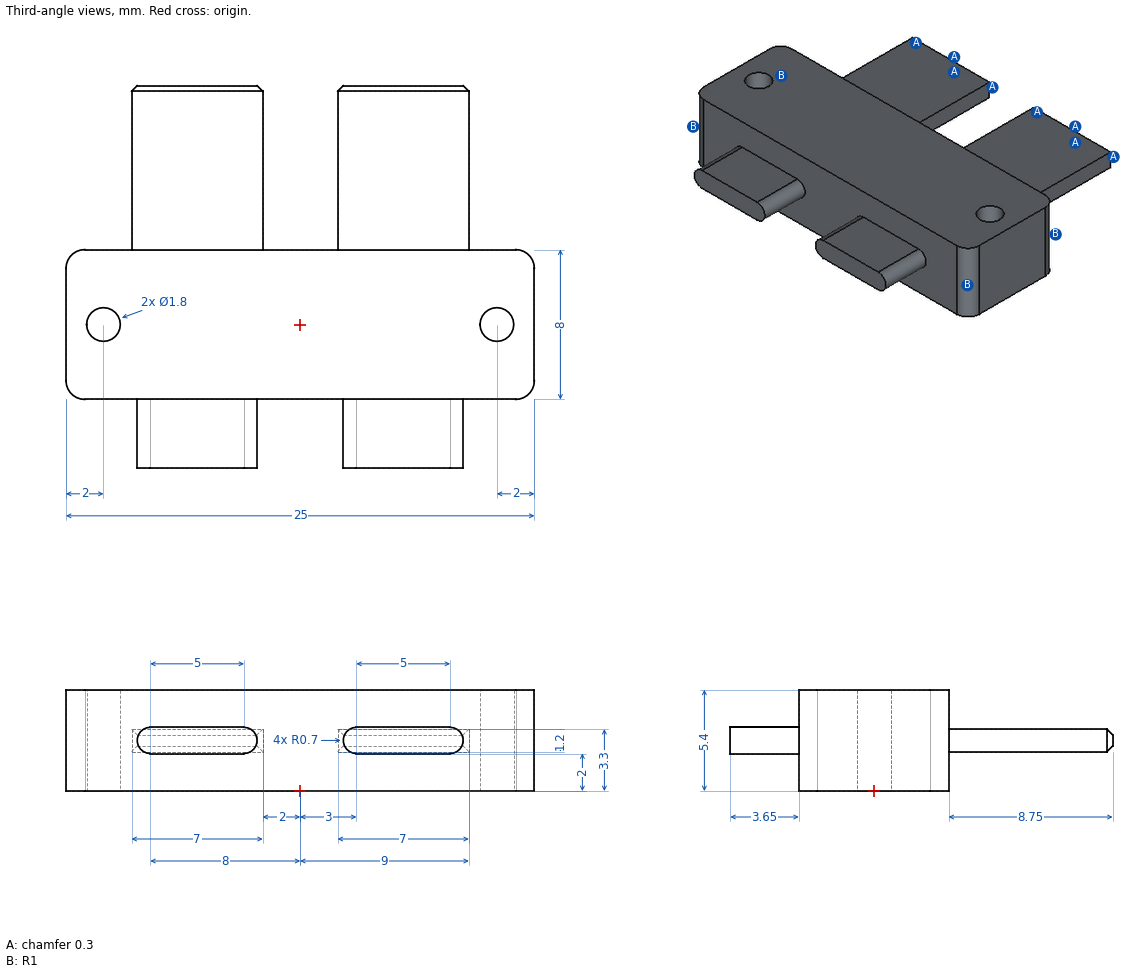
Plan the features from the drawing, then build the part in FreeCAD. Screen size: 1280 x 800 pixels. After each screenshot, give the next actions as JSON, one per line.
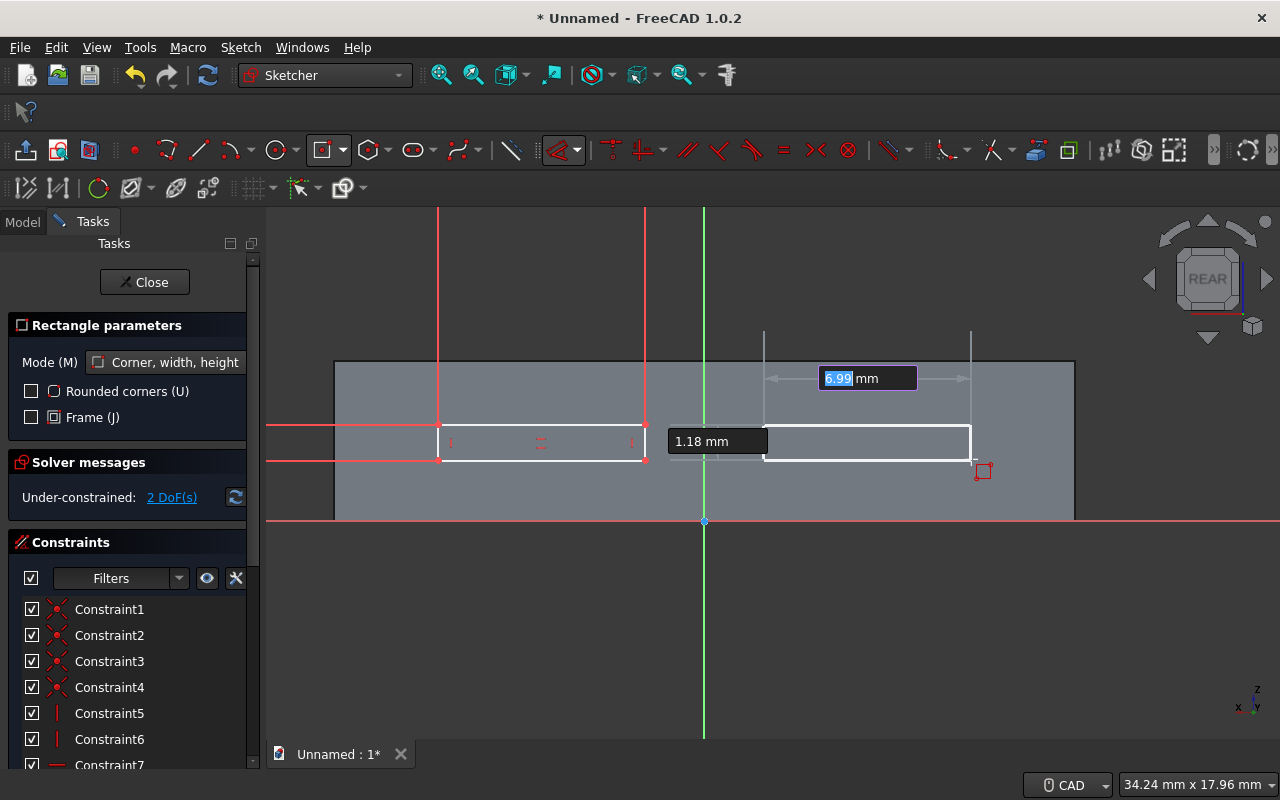
{"action": "type", "text": "7"}
{"action": "key", "text": "Tab"}
{"action": "type", "text": "1.2"}
{"action": "key", "text": "Return"}
{"action": "key", "text": "Escape"}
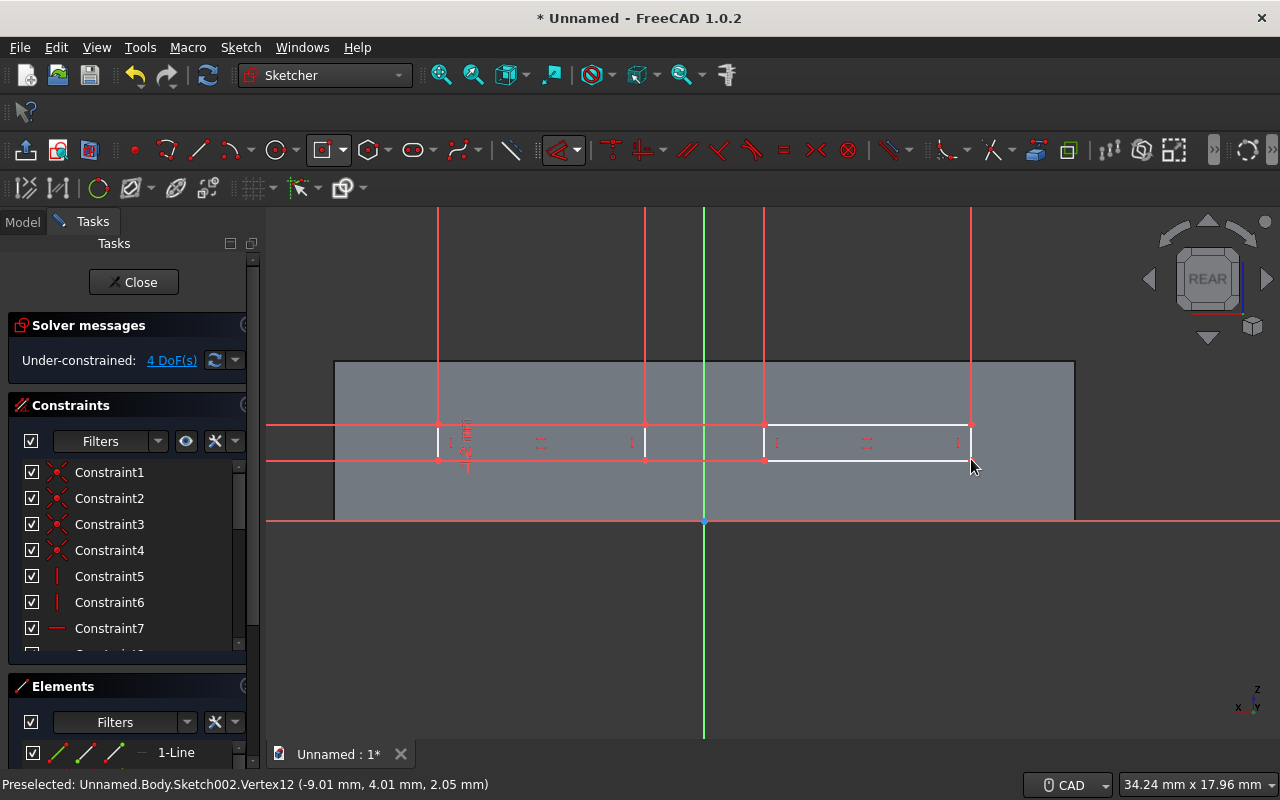
{"action": "left_click", "coordinate": [438, 425]}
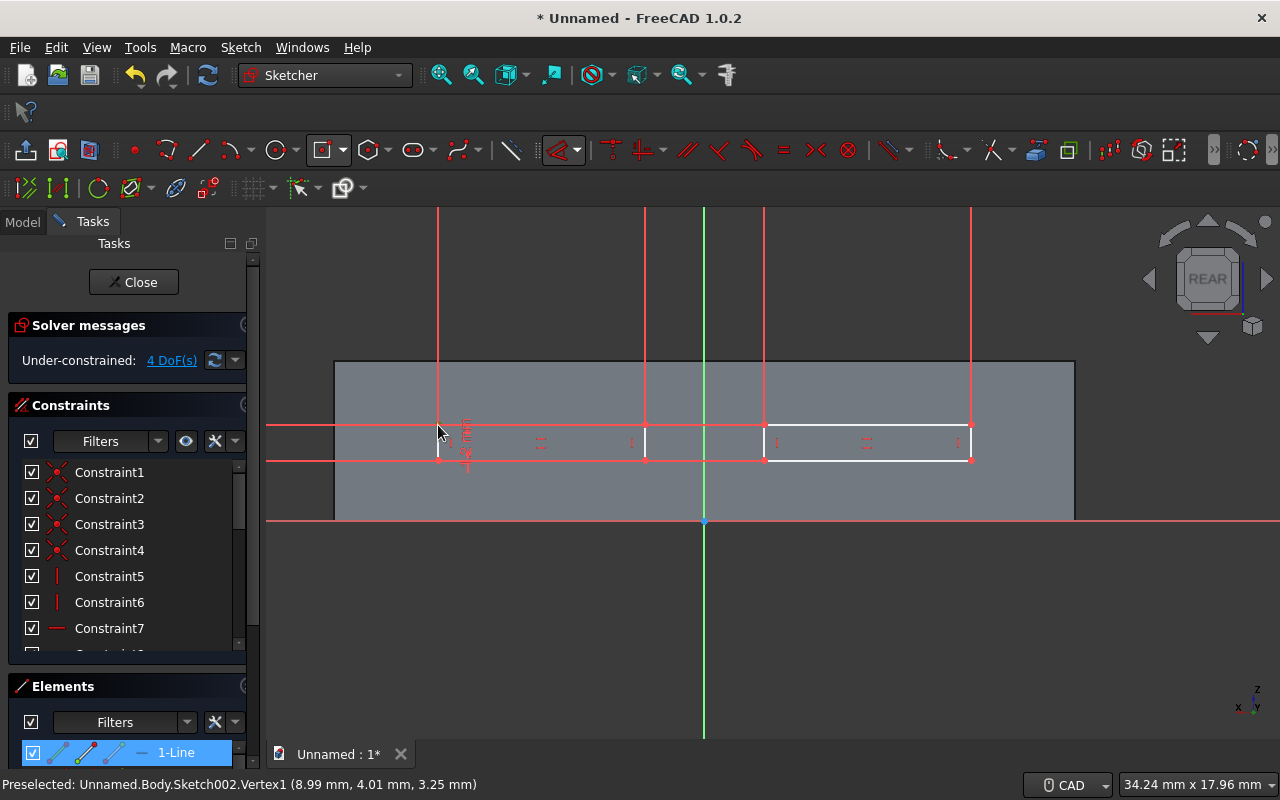
{"action": "left_click", "coordinate": [580, 150]}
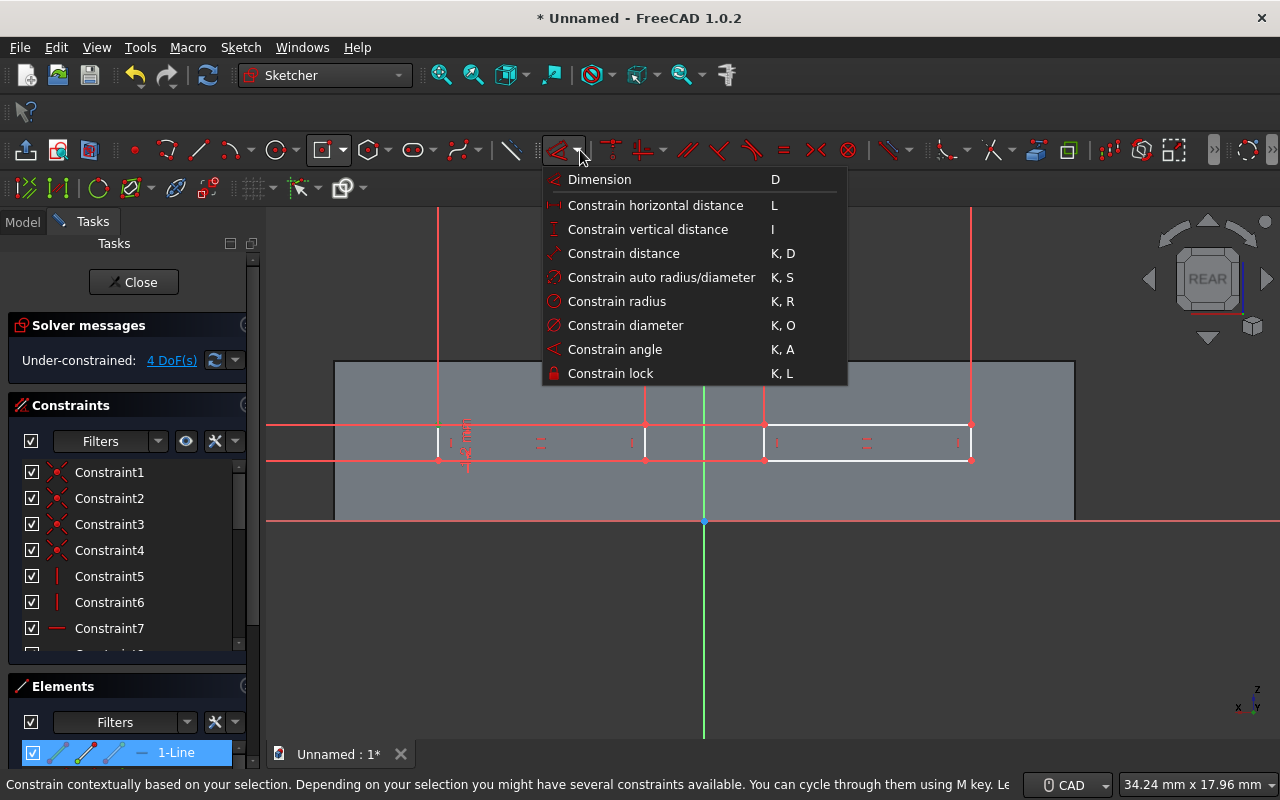
{"action": "left_click", "coordinate": [695, 205]}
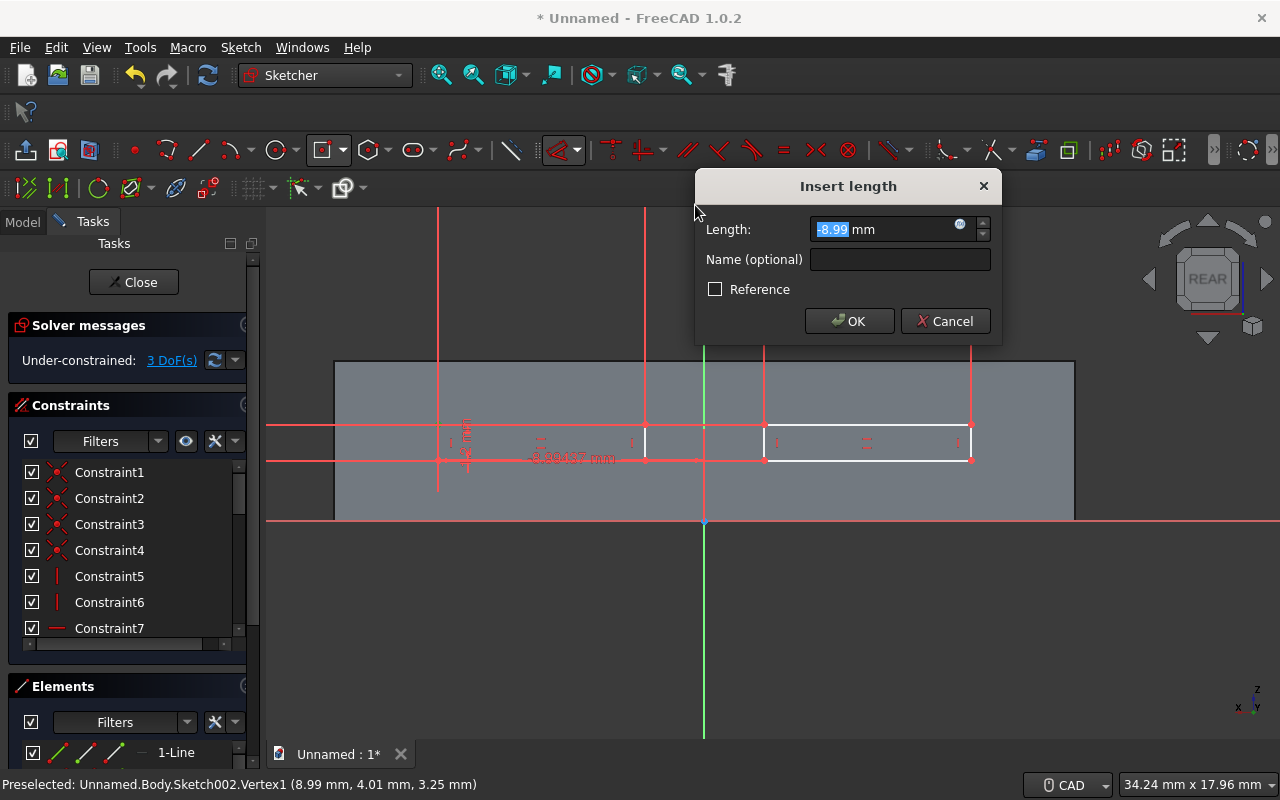
{"action": "type", "text": "-9"}
{"action": "key", "text": "Return"}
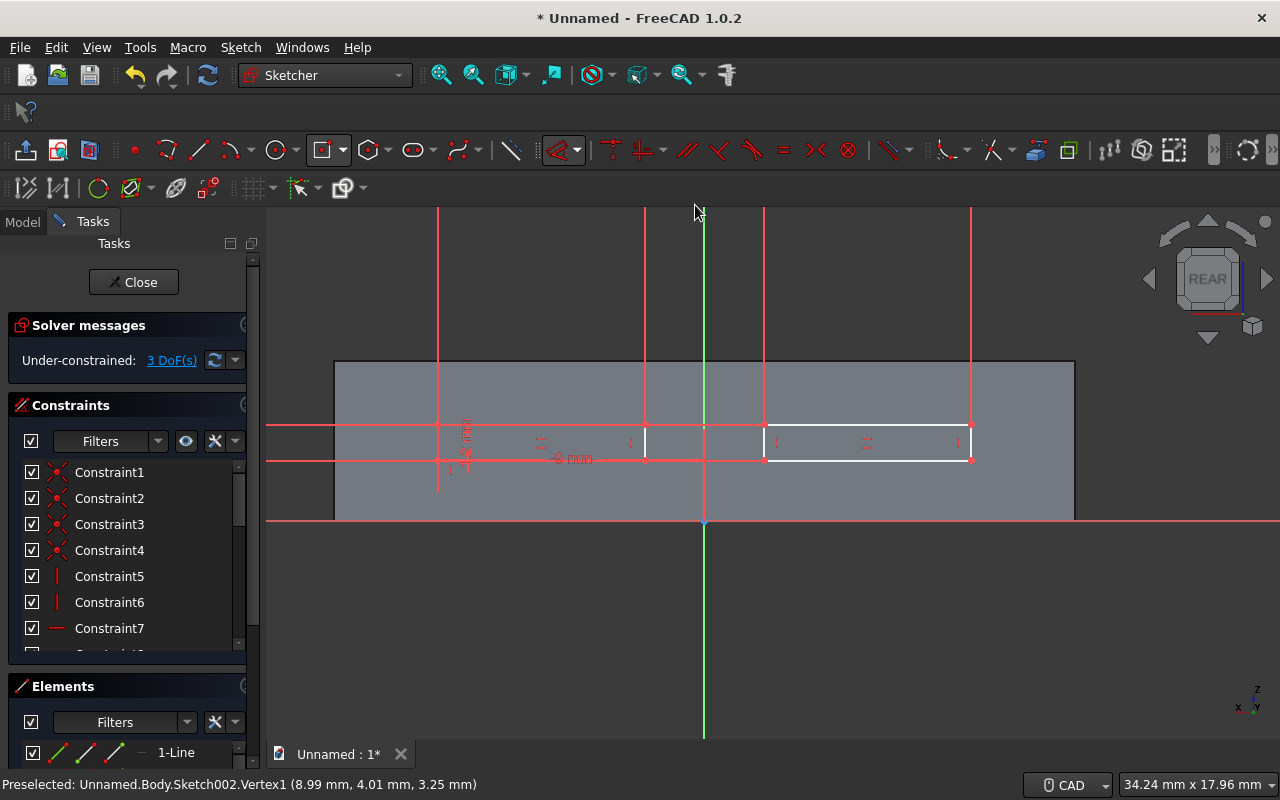
{"action": "left_click", "coordinate": [764, 425]}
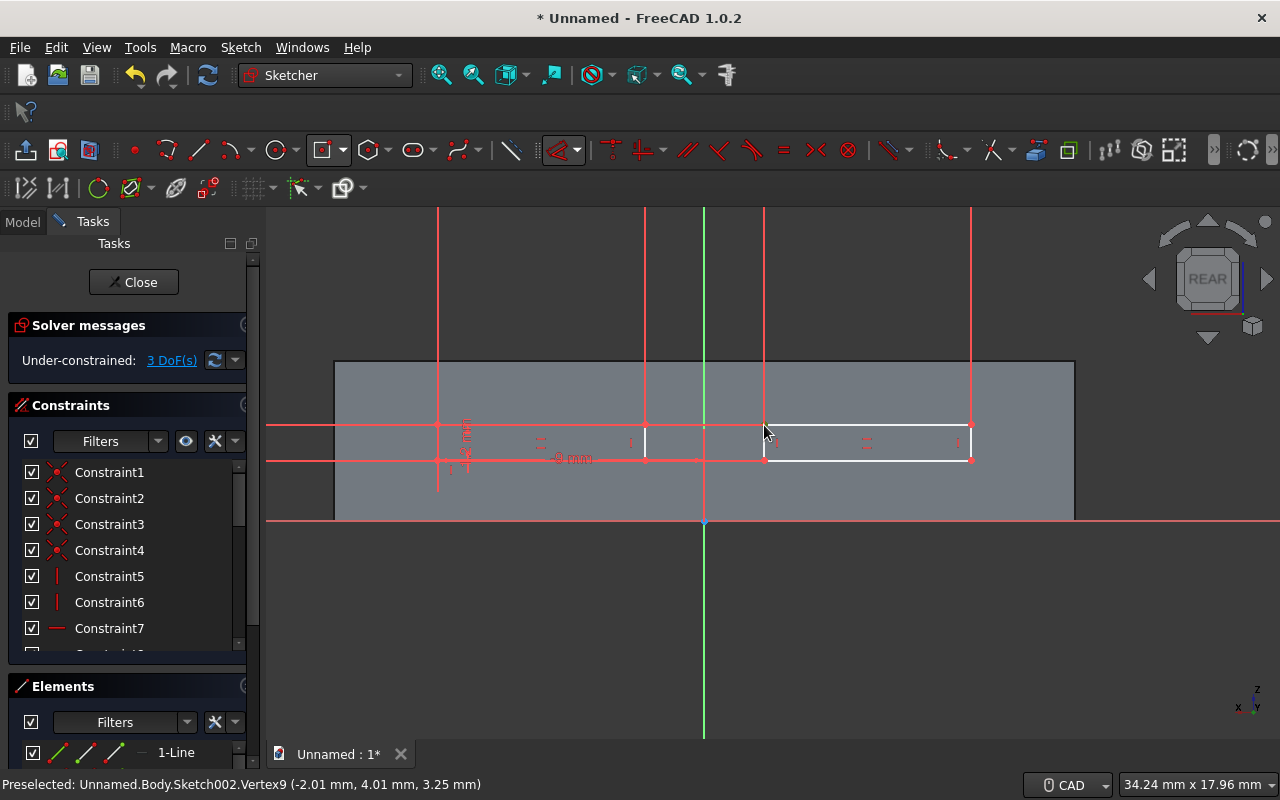
{"action": "left_click", "coordinate": [580, 150]}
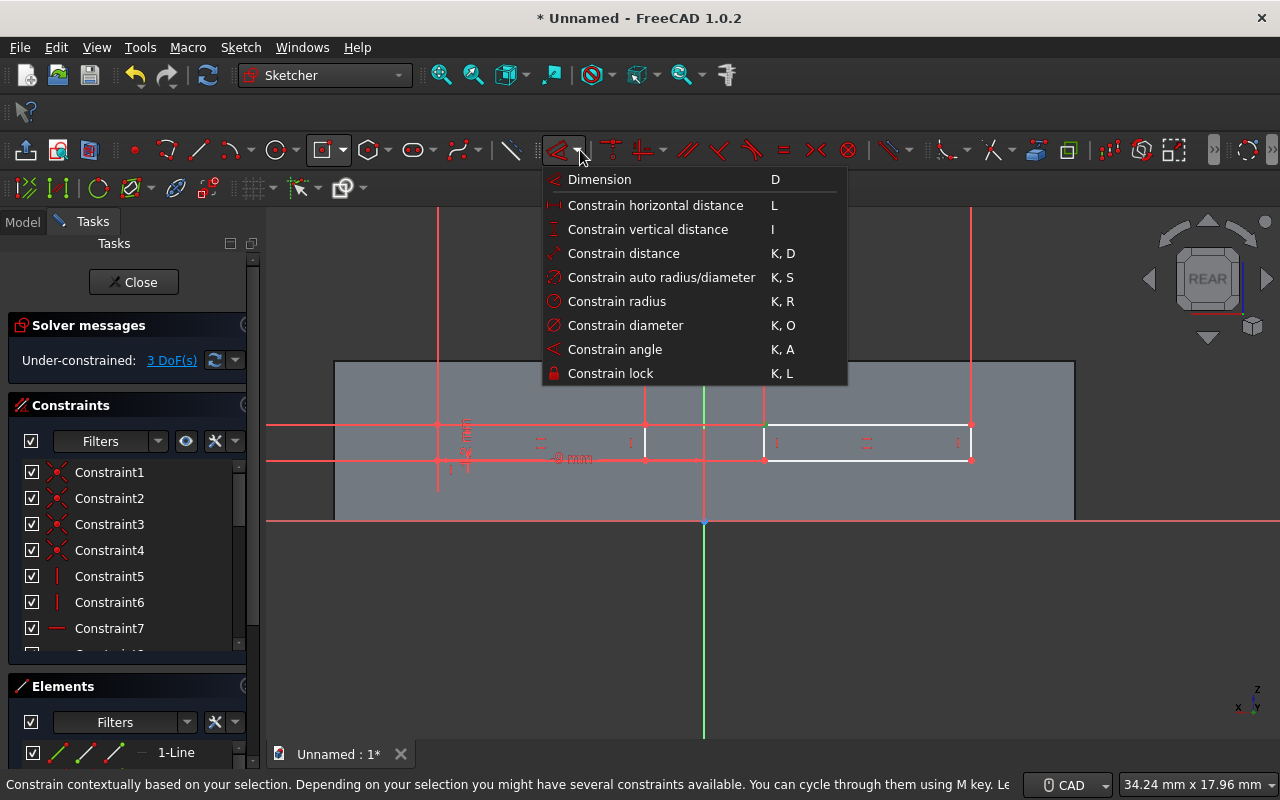
{"action": "left_click", "coordinate": [695, 205]}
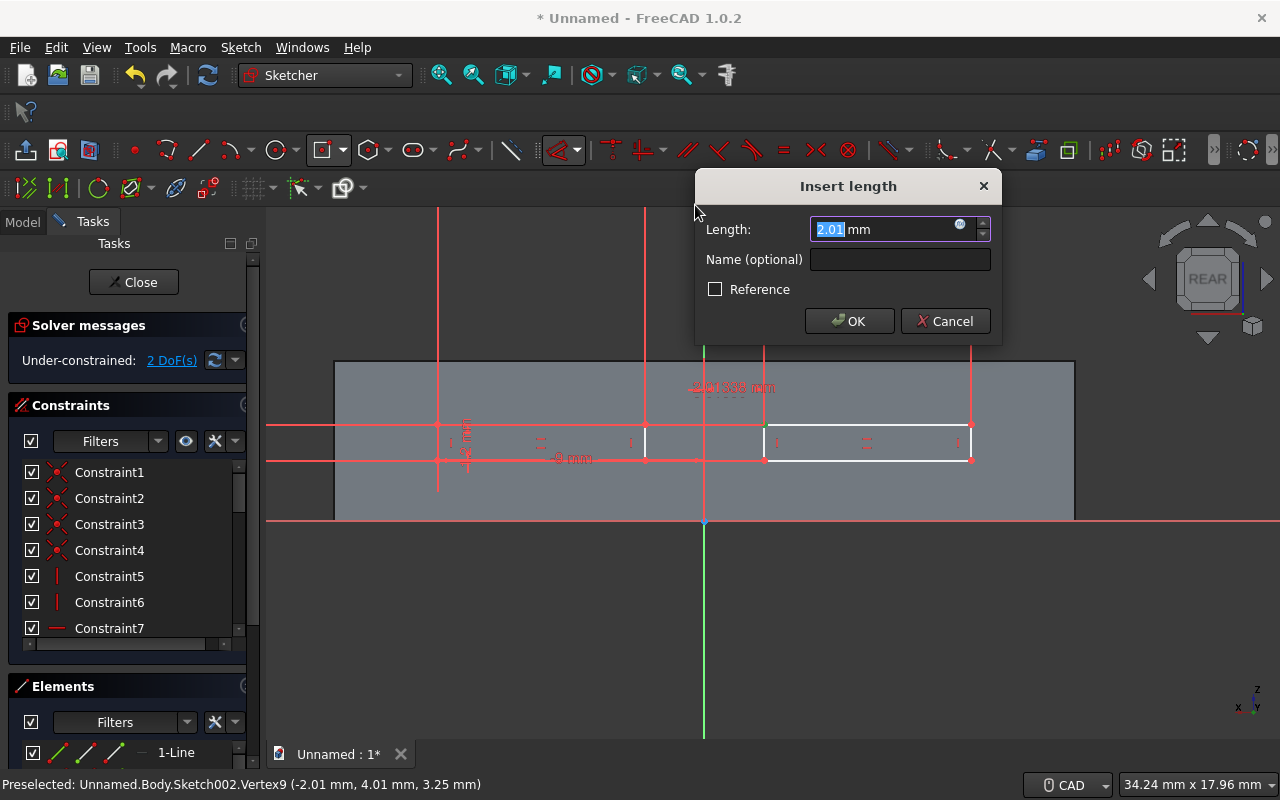
{"action": "type", "text": "2"}
{"action": "key", "text": "Return"}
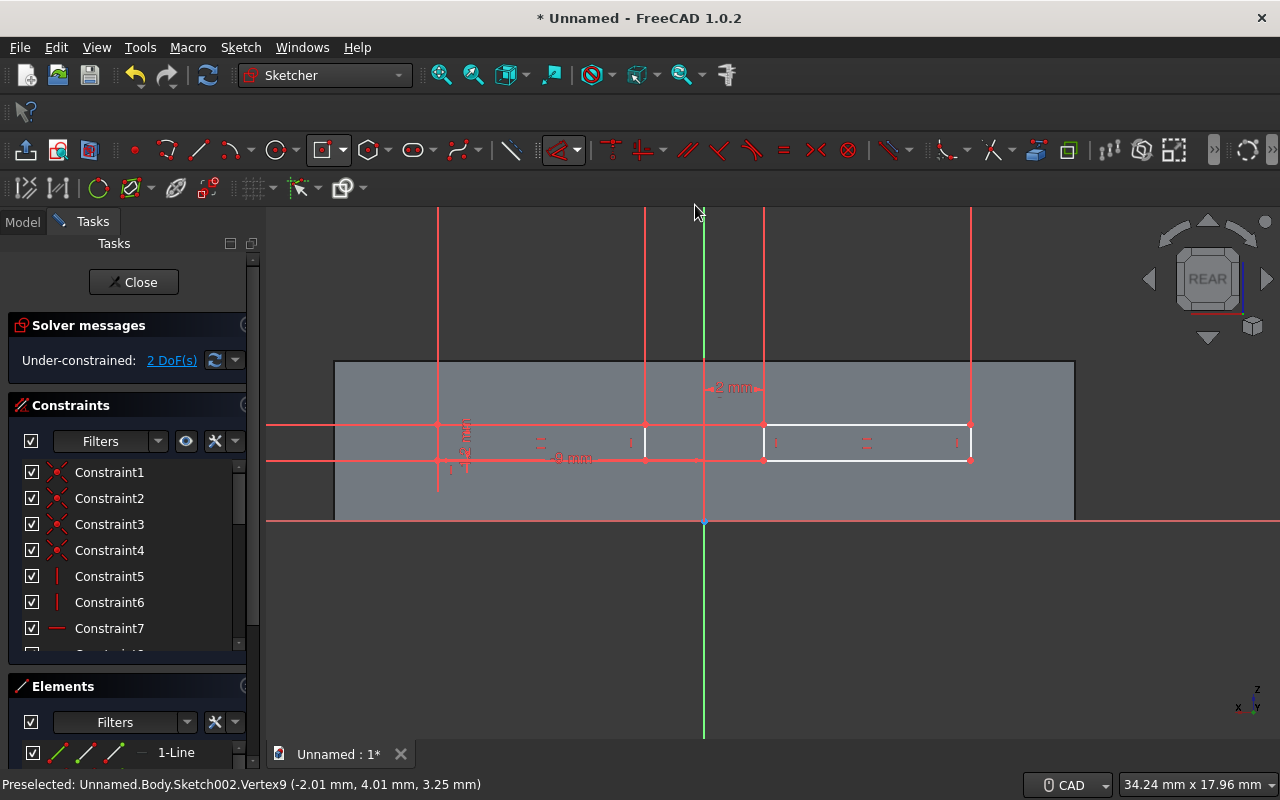
{"action": "left_click", "coordinate": [438, 425]}